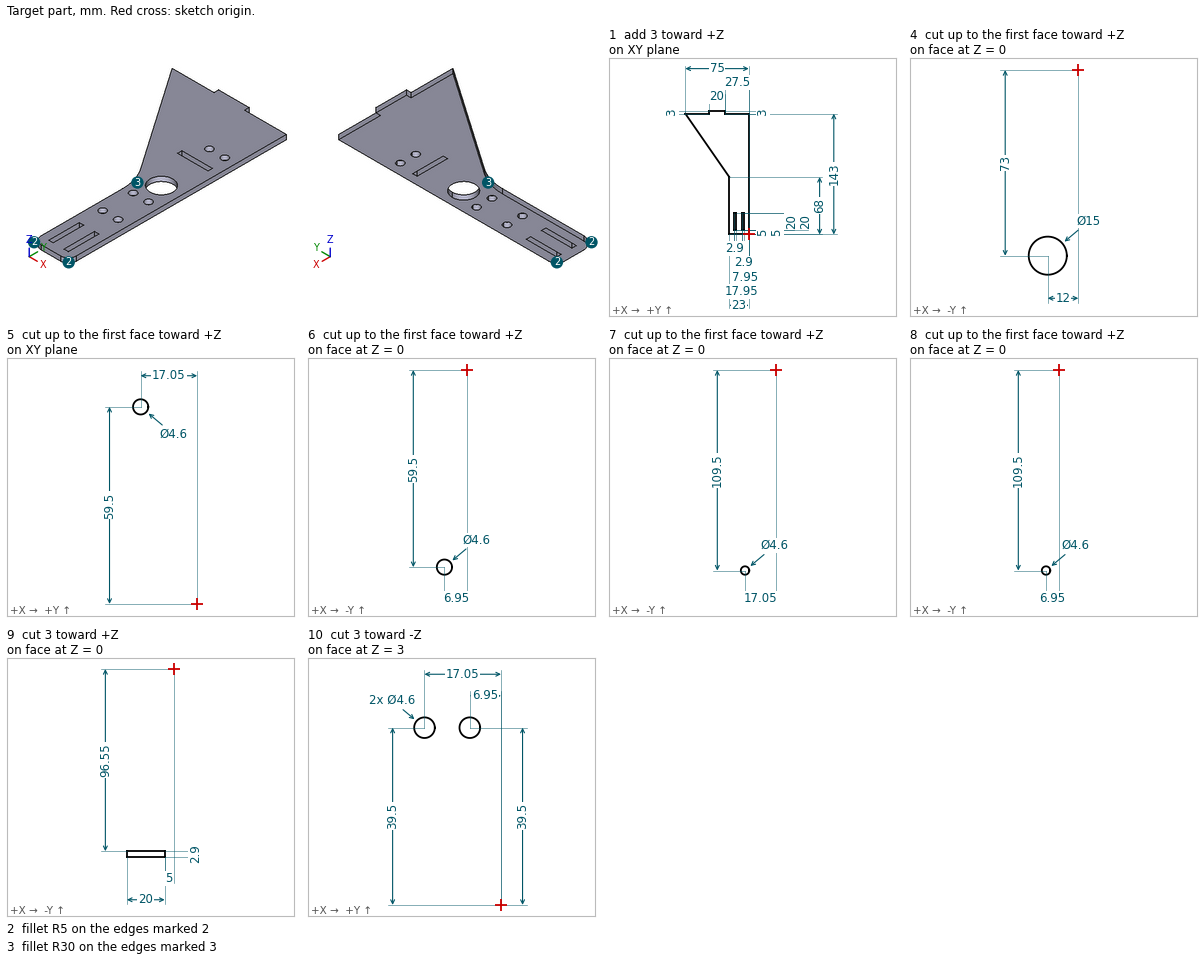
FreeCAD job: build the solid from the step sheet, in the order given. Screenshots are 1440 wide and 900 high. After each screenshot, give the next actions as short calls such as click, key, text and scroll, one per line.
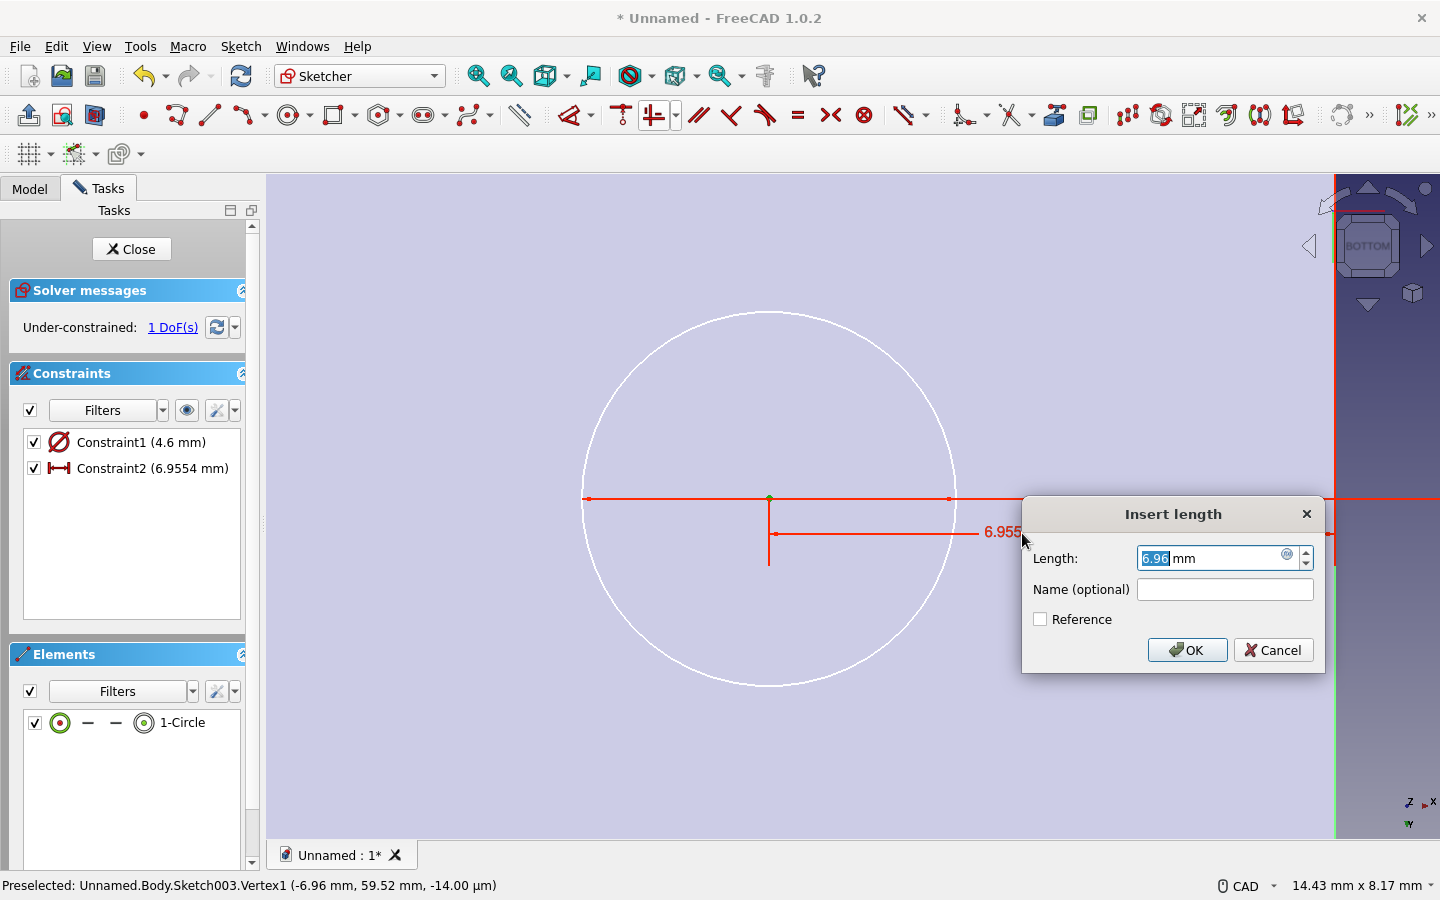
text(6.95)
key(Return)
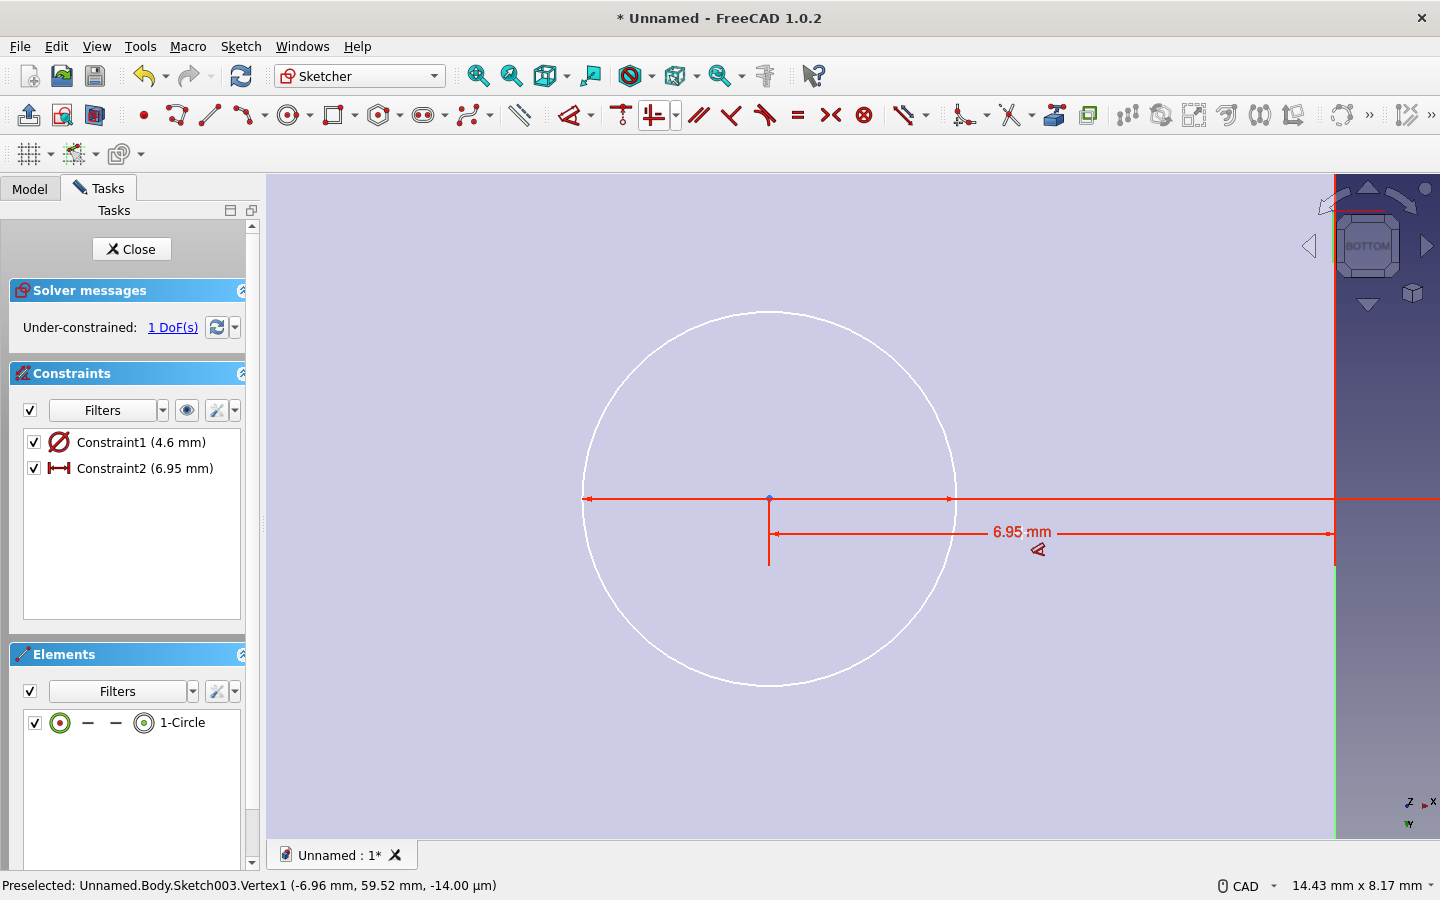
click(769, 499)
click(735, 351)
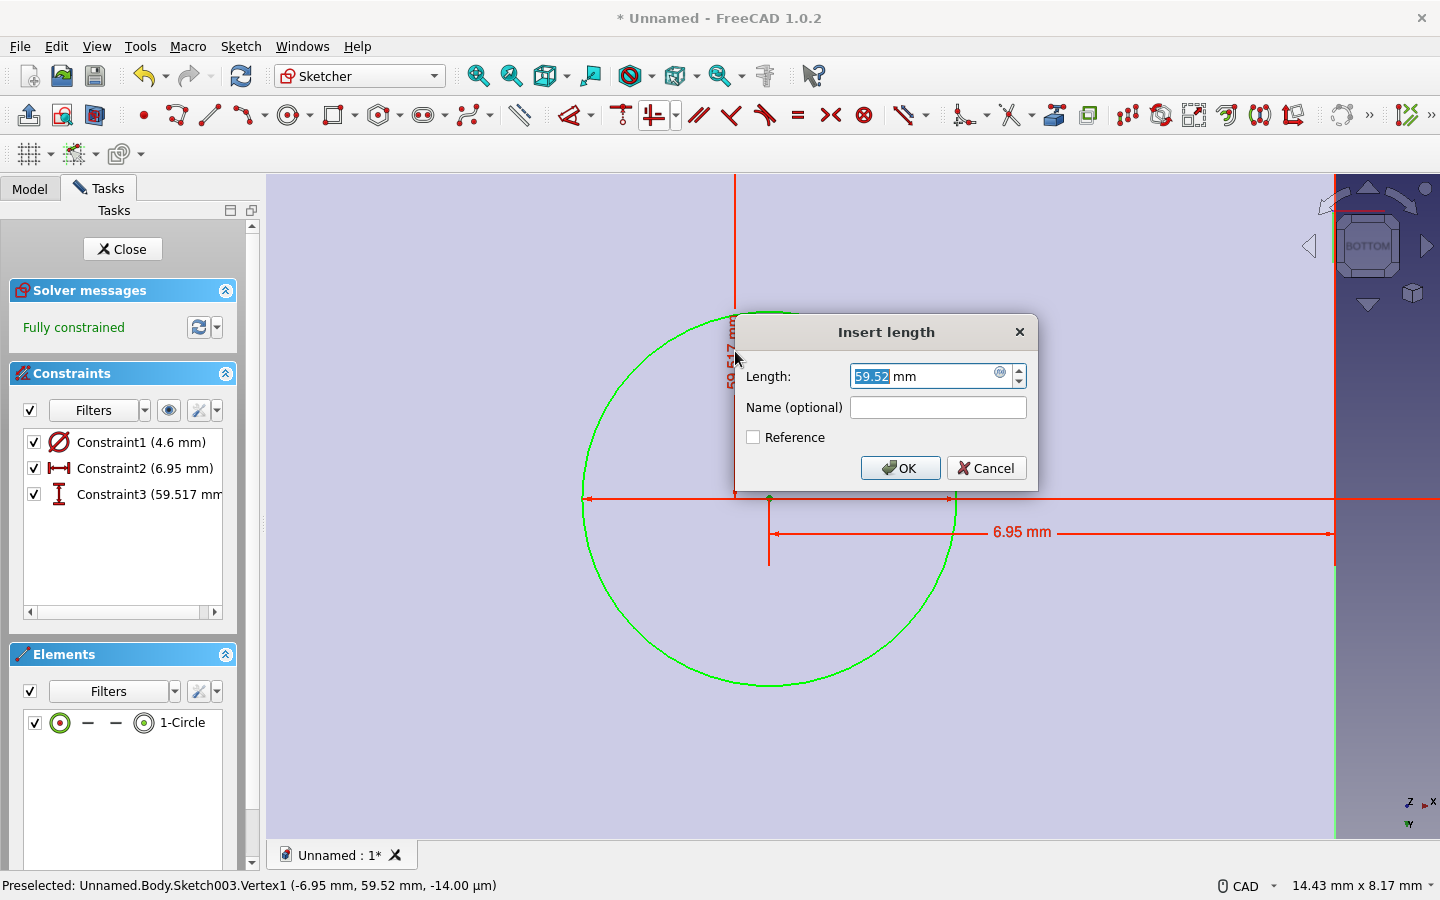
text(59.5)
key(Return)
key(Escape)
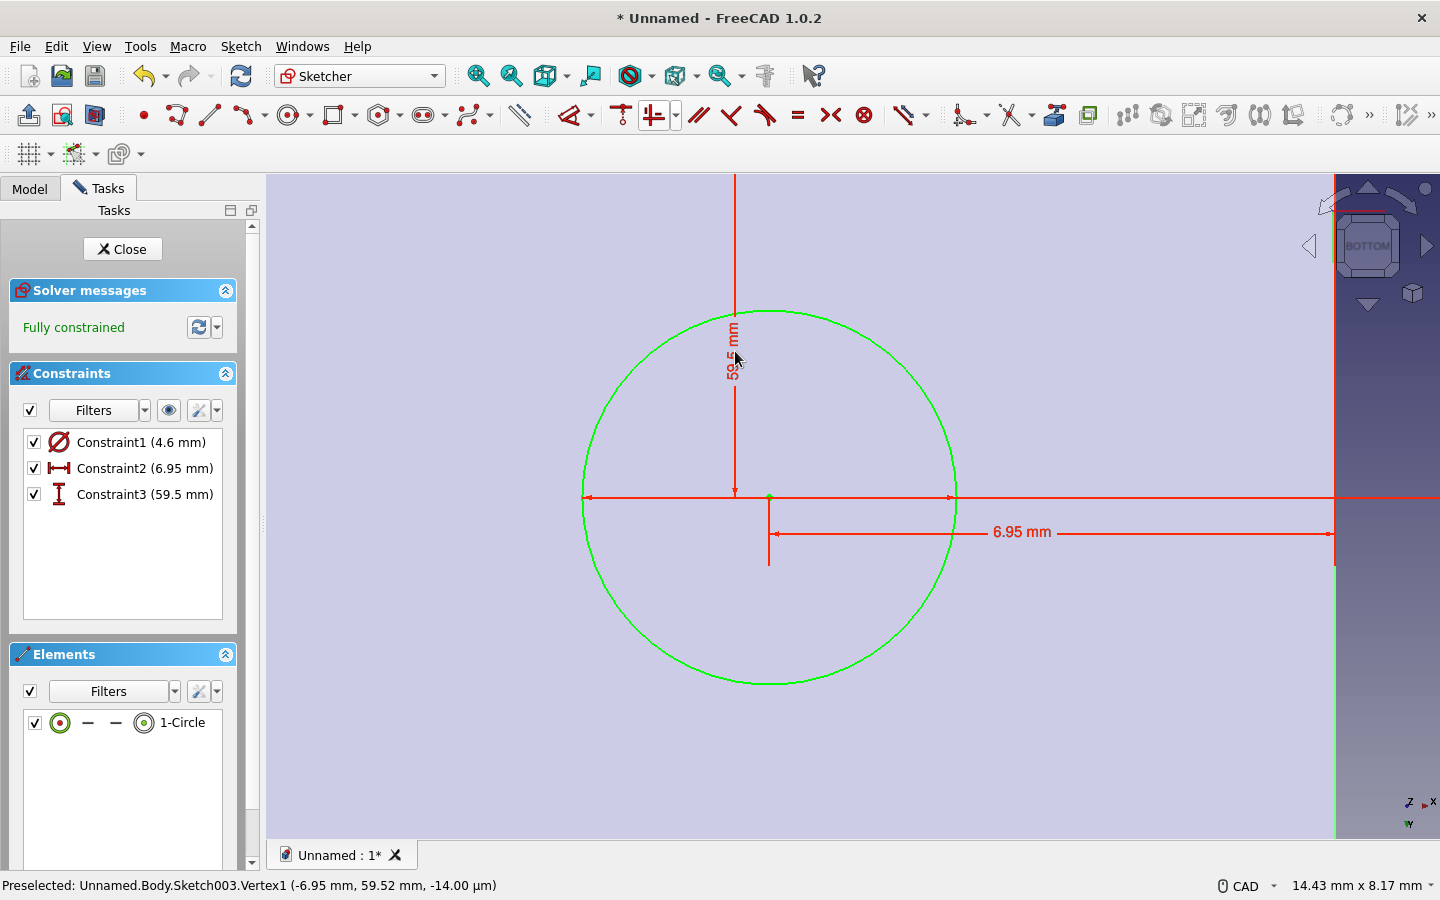
click(123, 249)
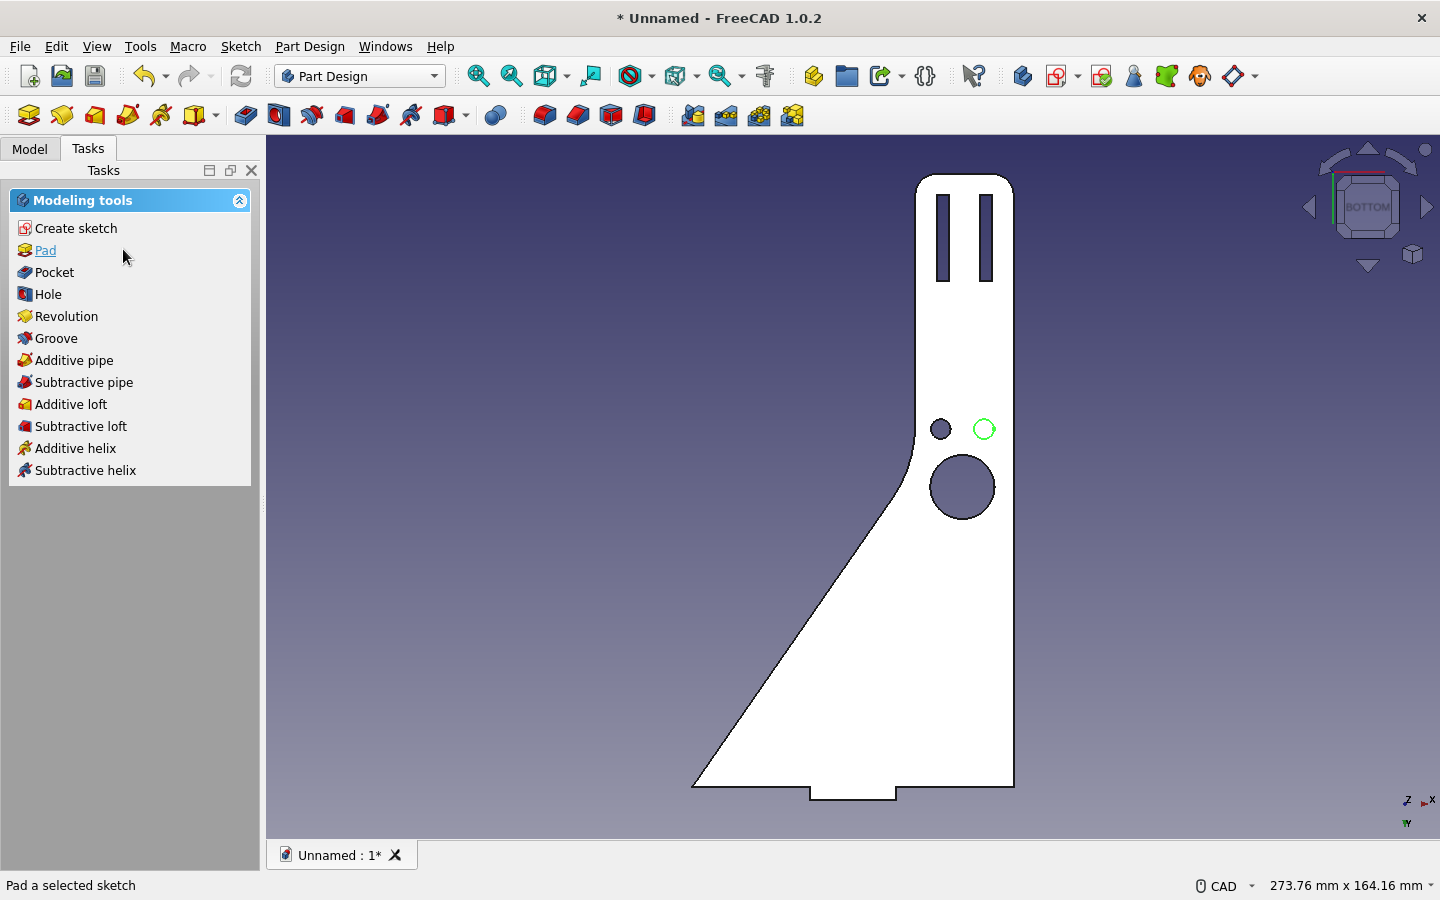
click(246, 116)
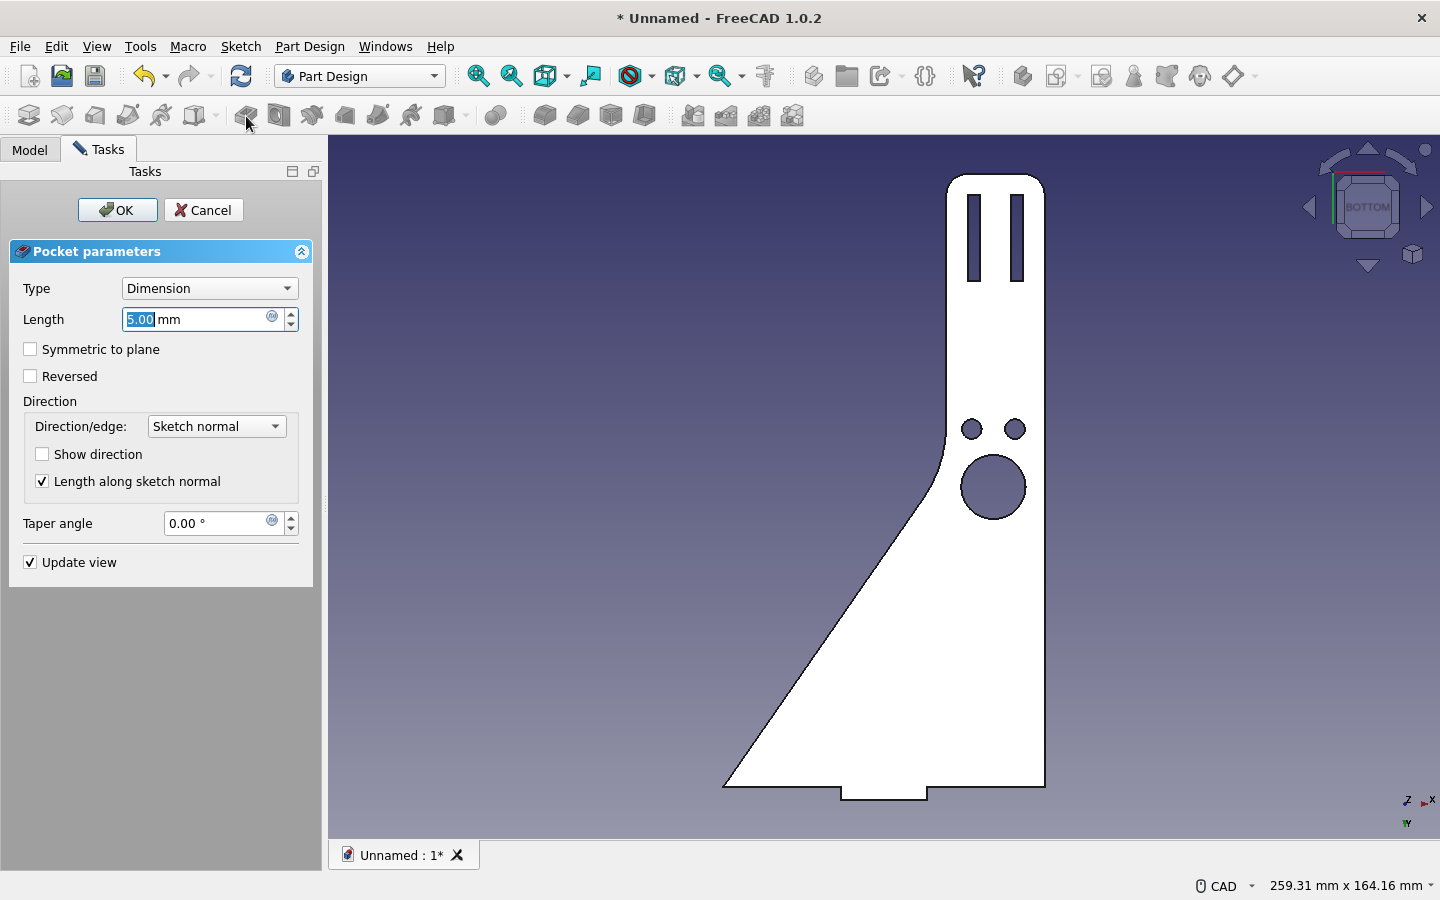
click(210, 288)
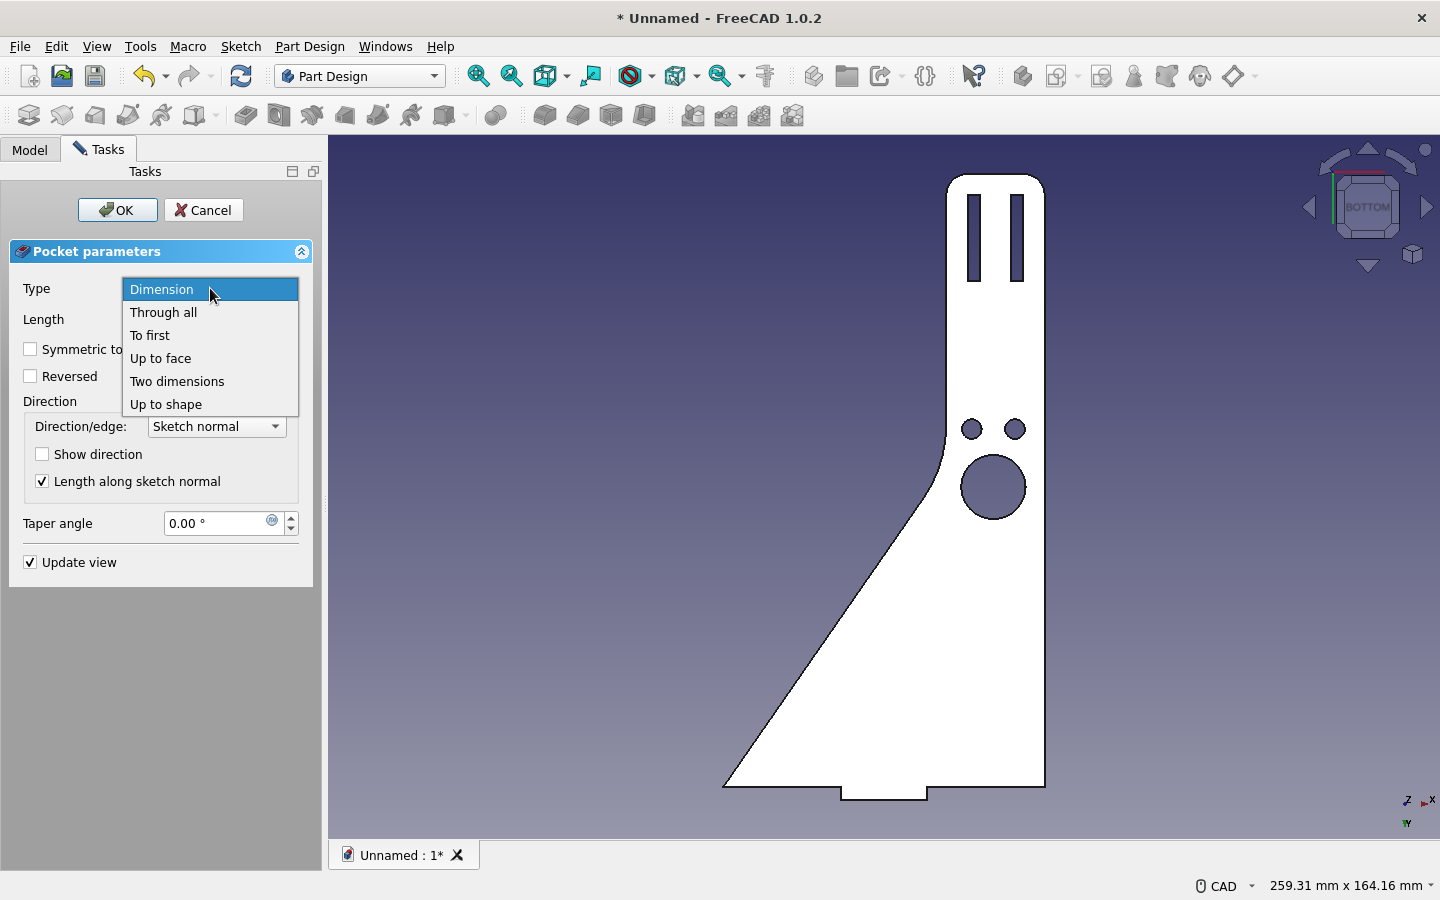
click(208, 336)